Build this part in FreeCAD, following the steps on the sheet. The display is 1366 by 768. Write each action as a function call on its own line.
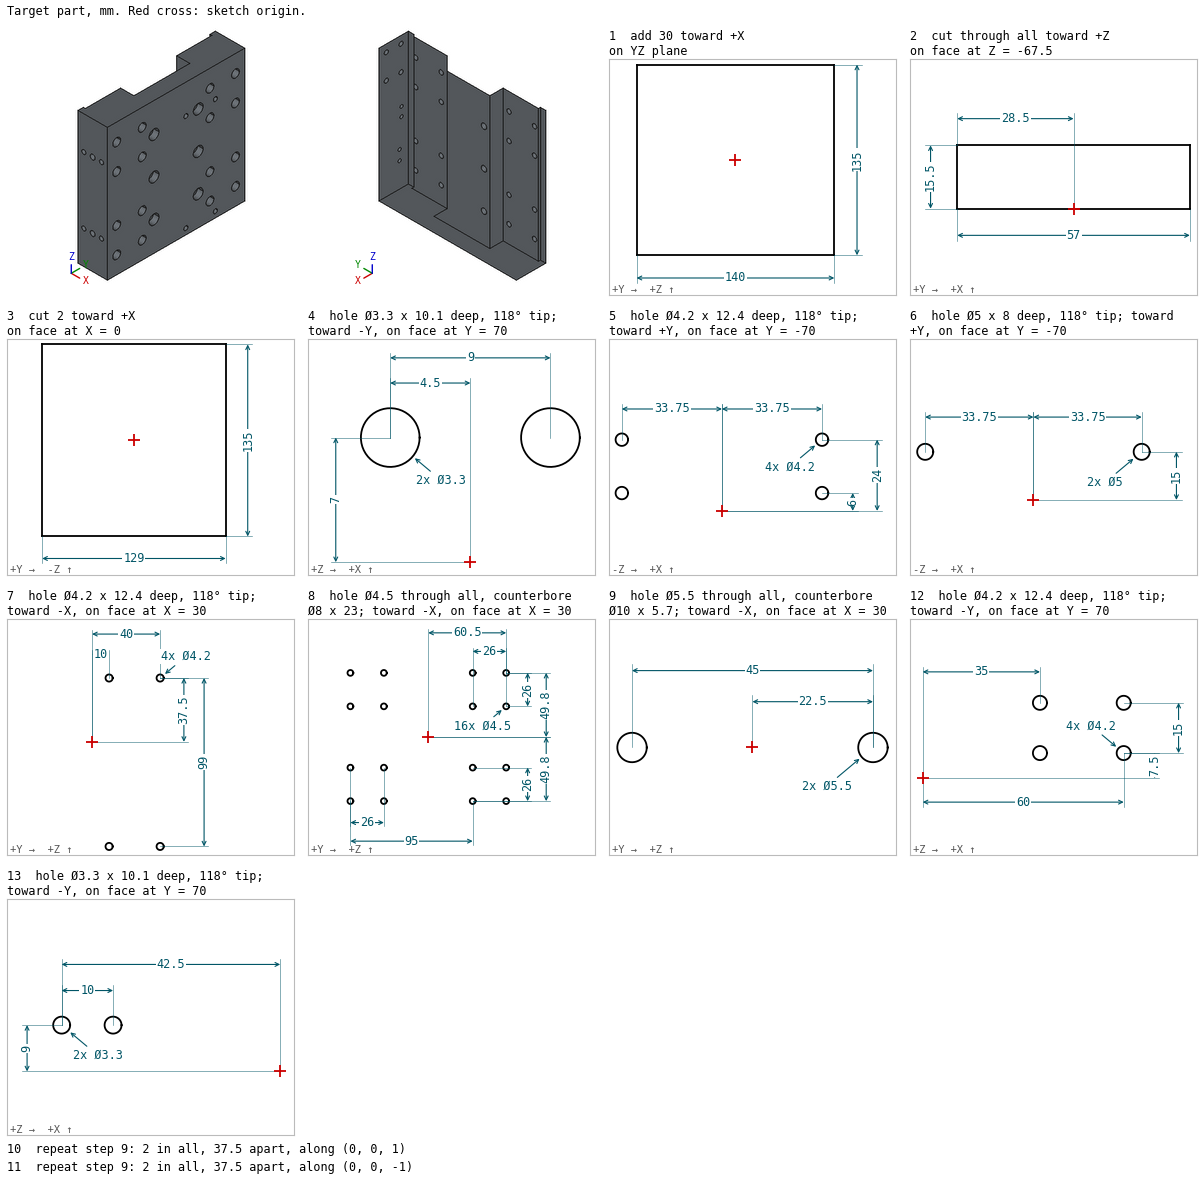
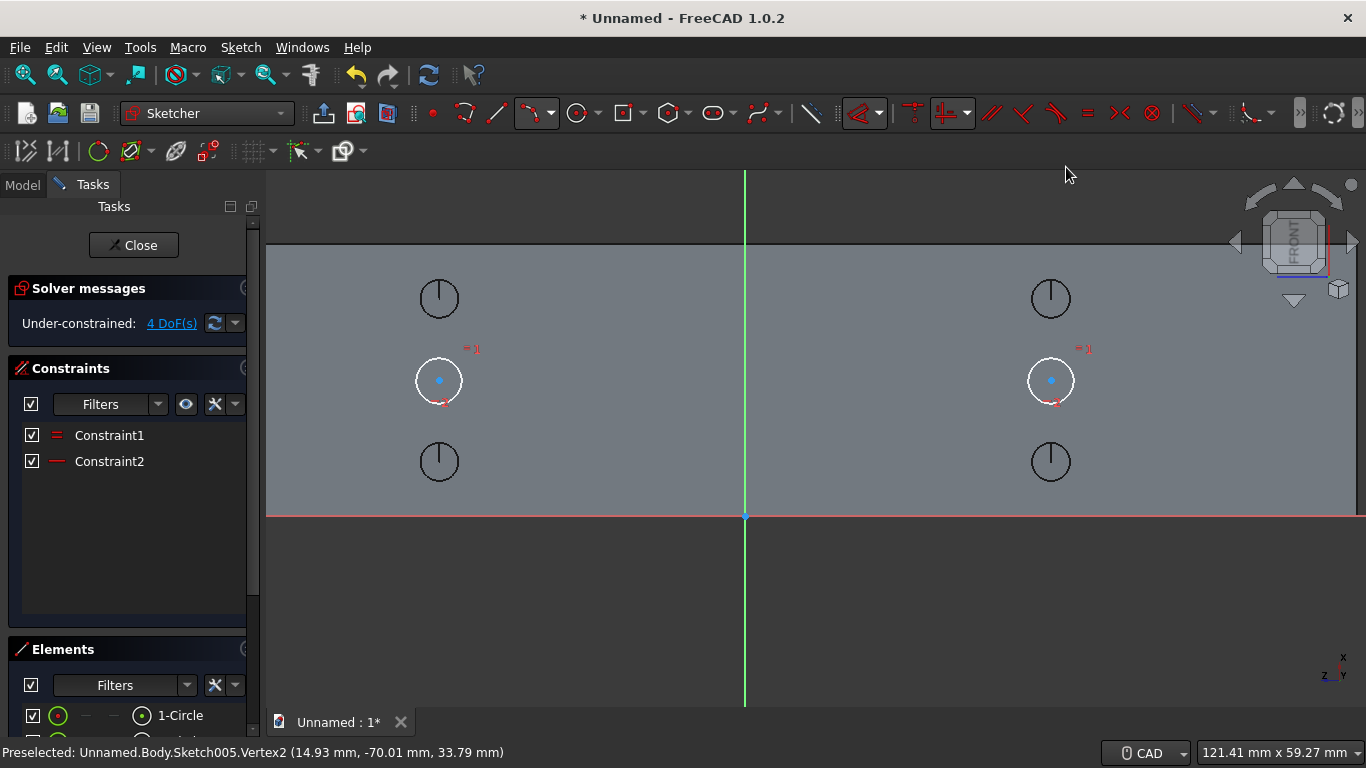
click(1067, 365)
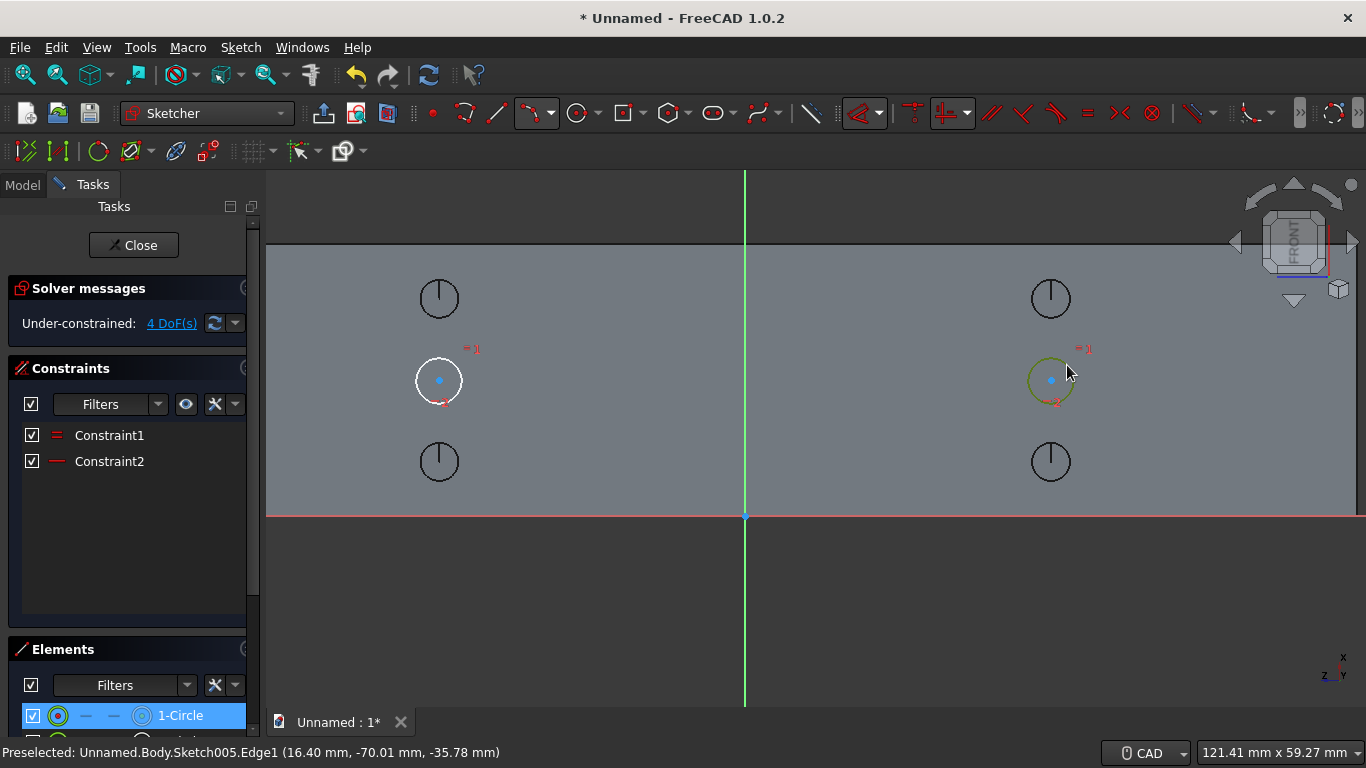
key(k)
key(o)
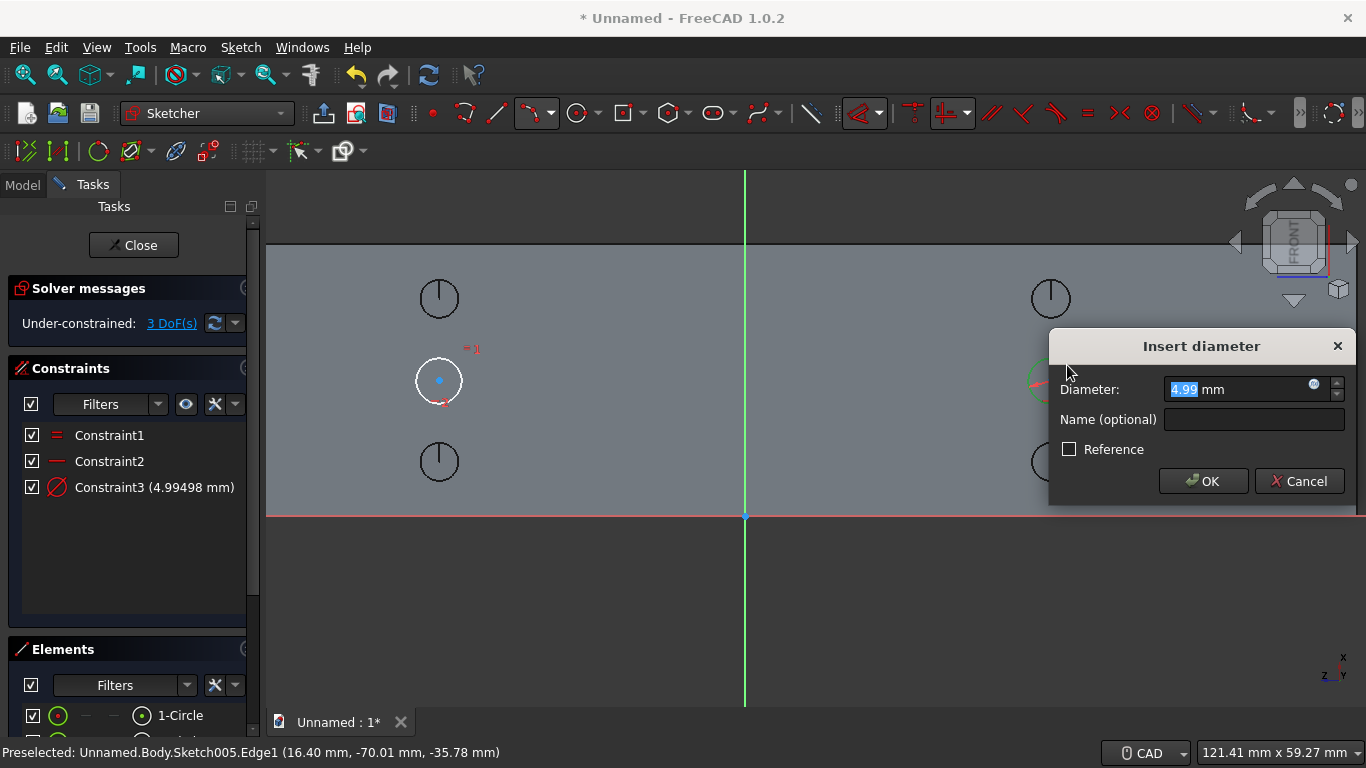
text(5)
key(Return)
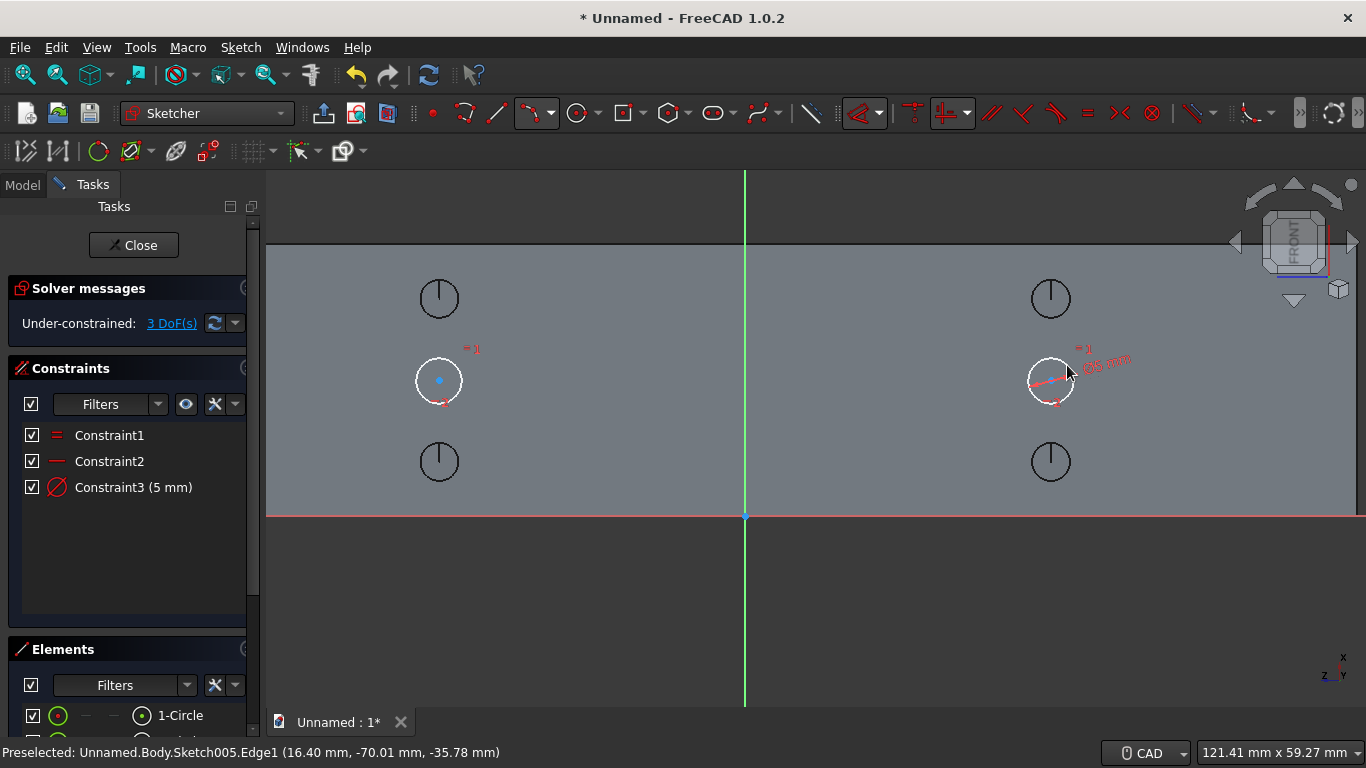
click(1051, 381)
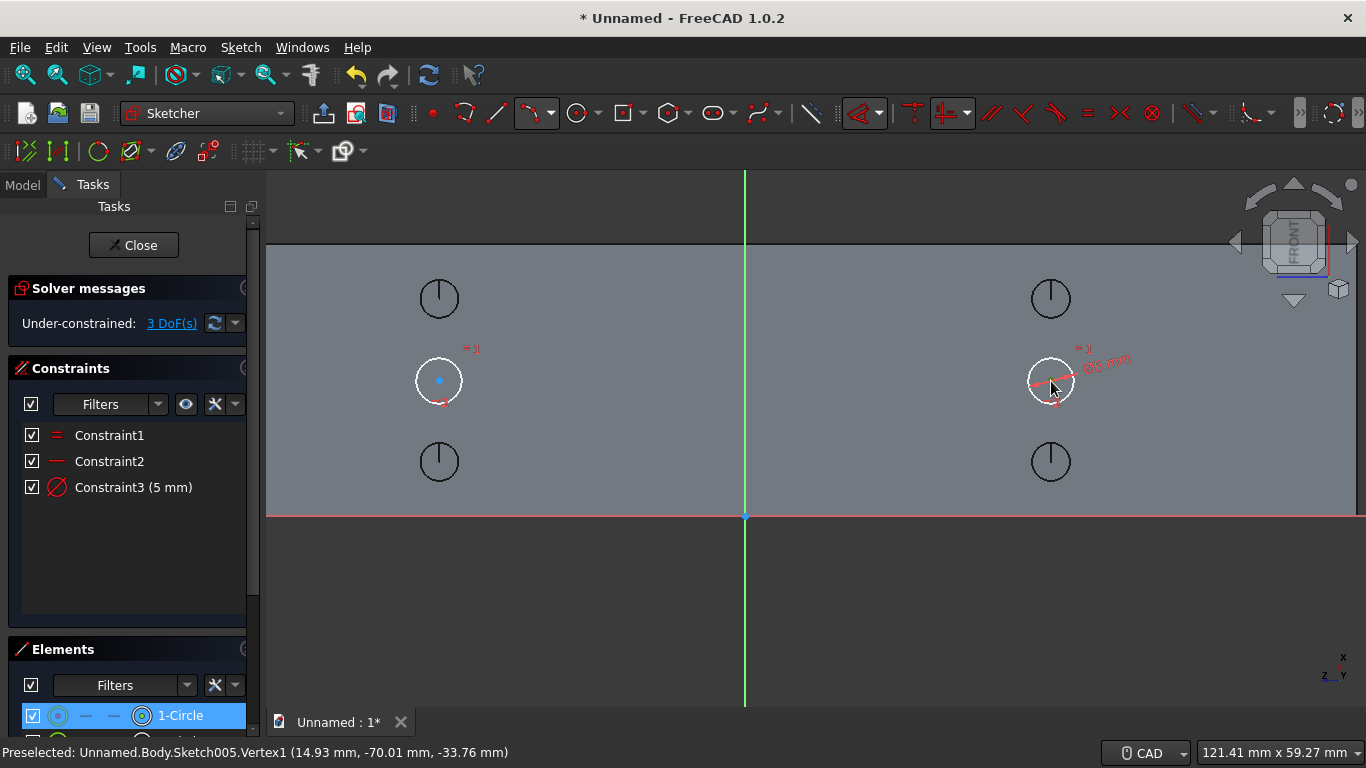
click(882, 114)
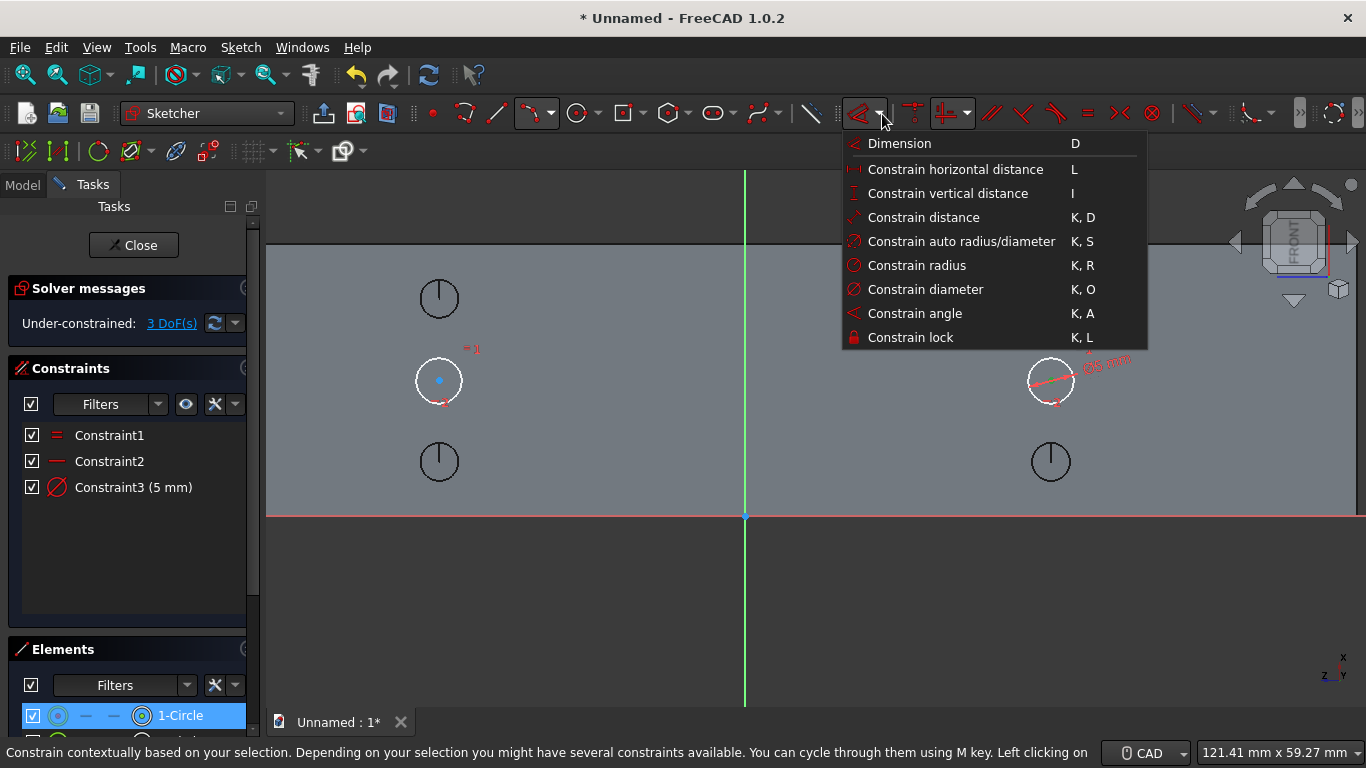
click(995, 193)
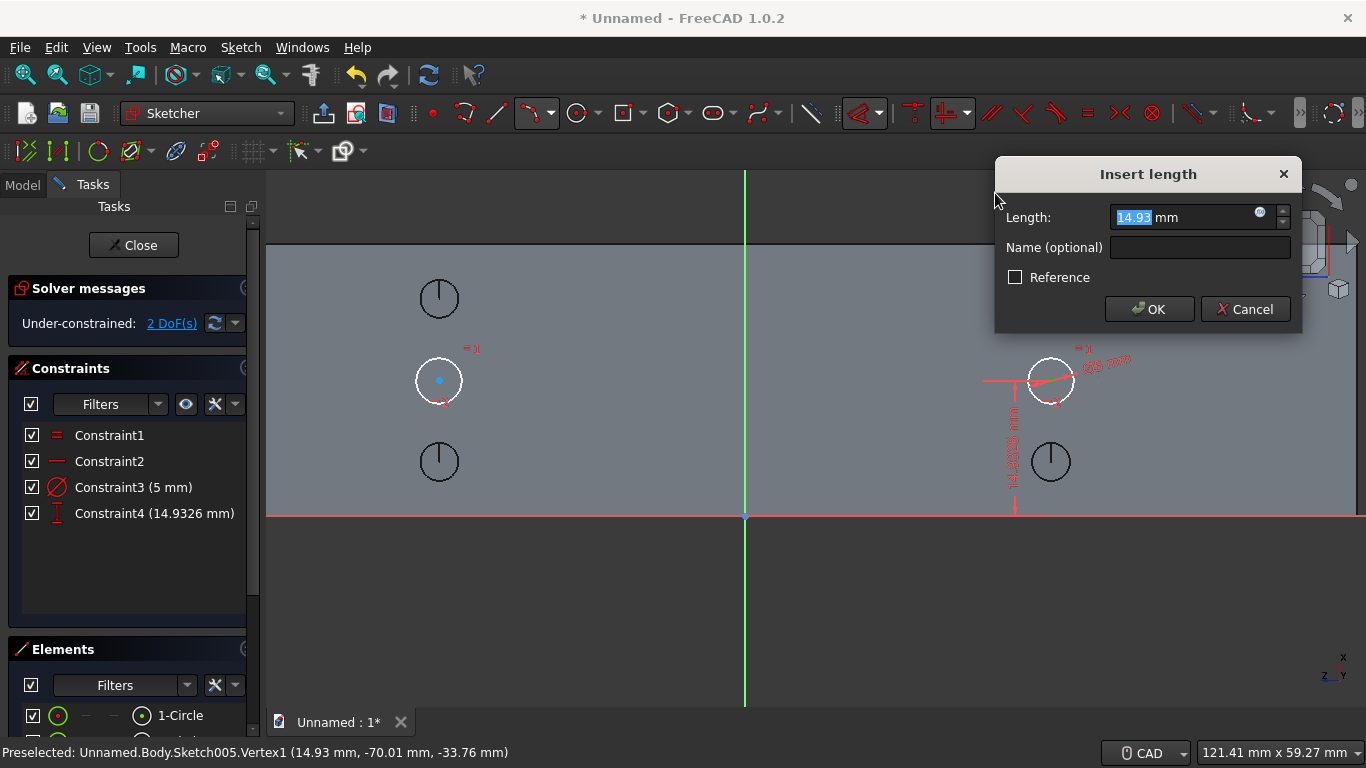
text(15)
key(Return)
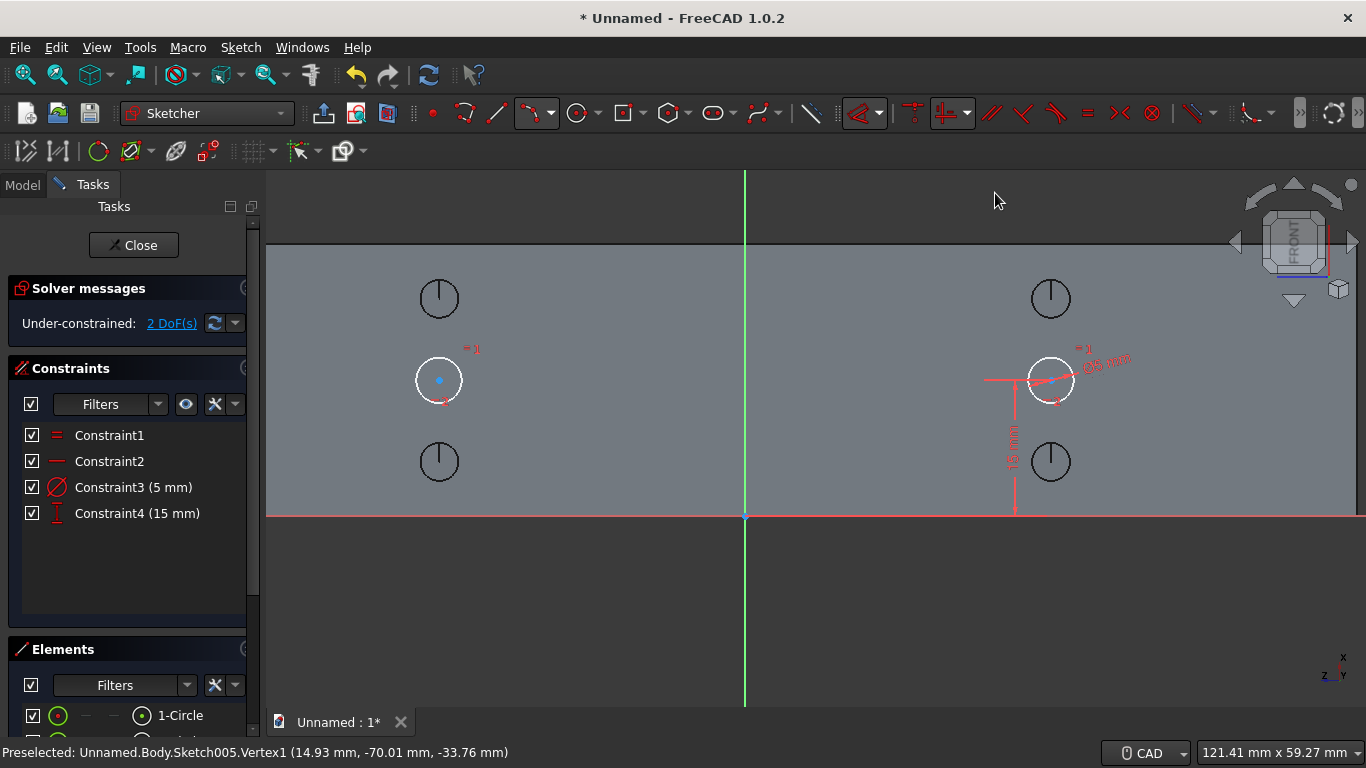
click(1051, 380)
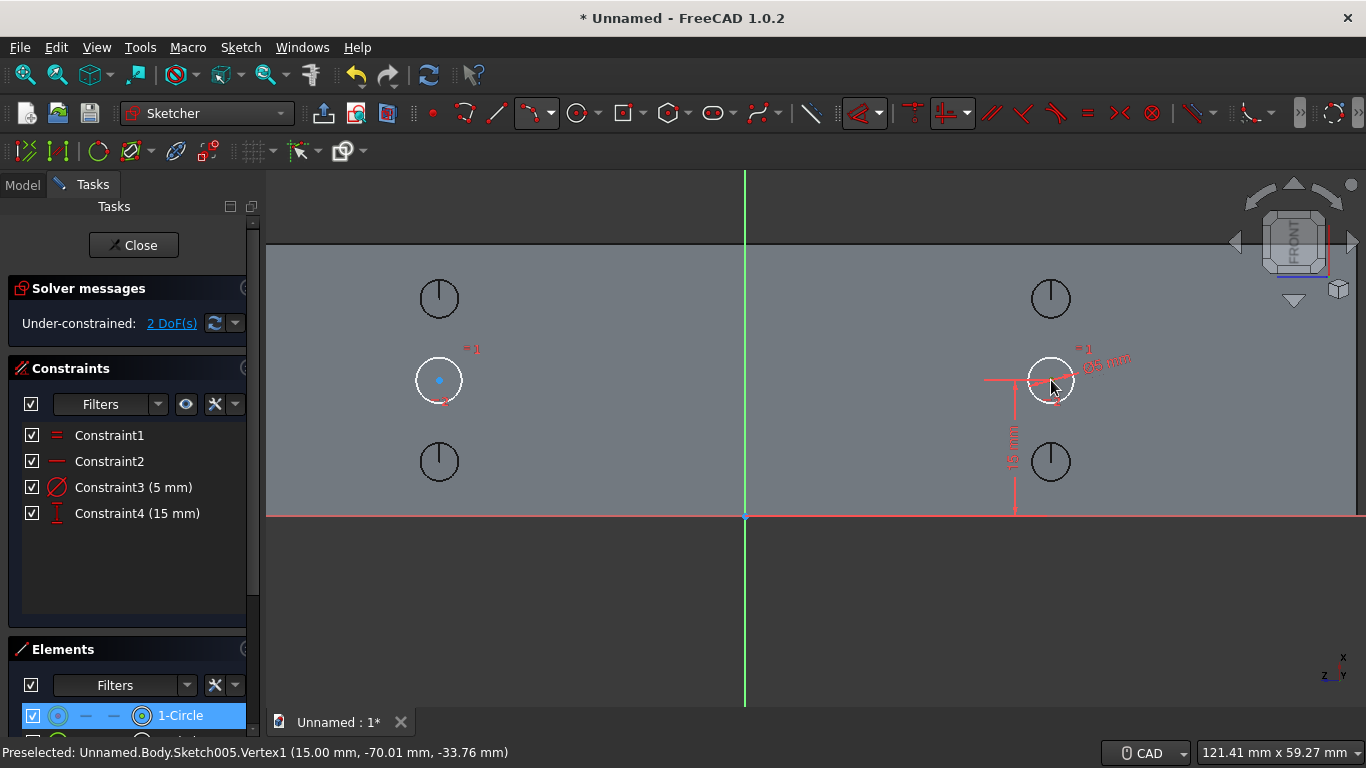
click(882, 114)